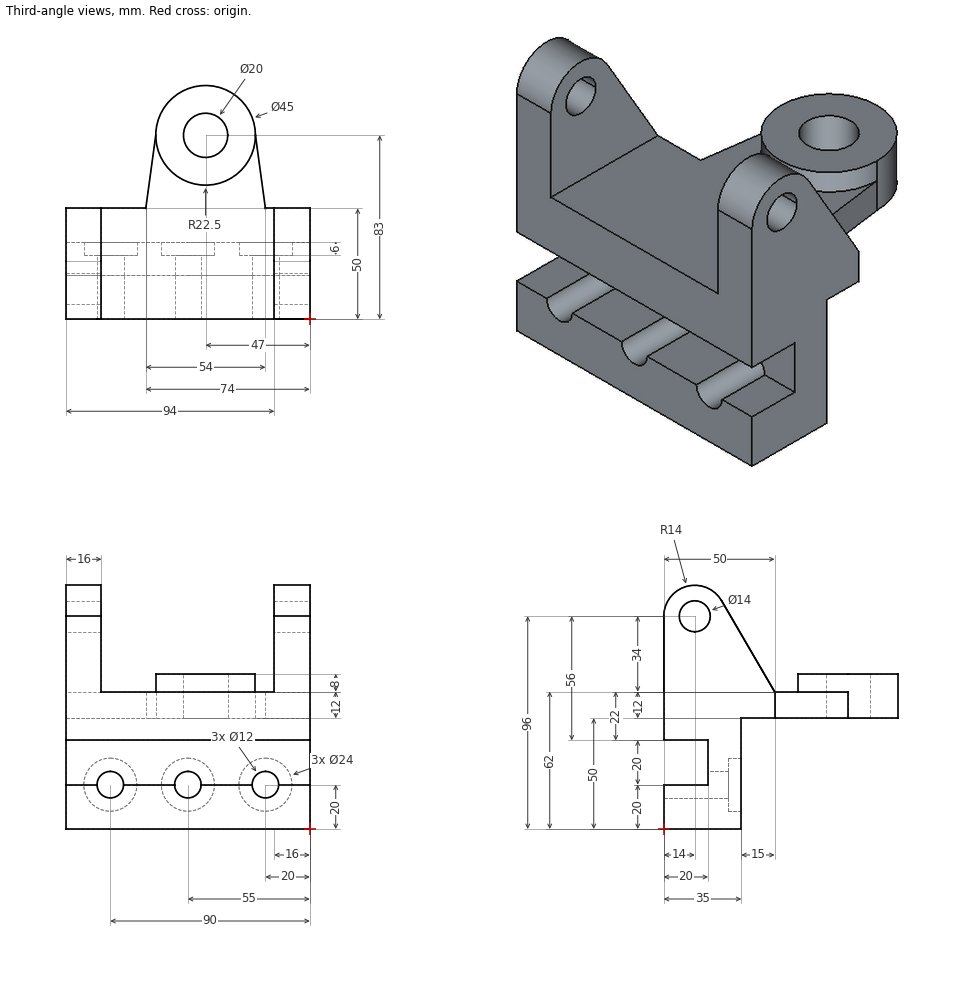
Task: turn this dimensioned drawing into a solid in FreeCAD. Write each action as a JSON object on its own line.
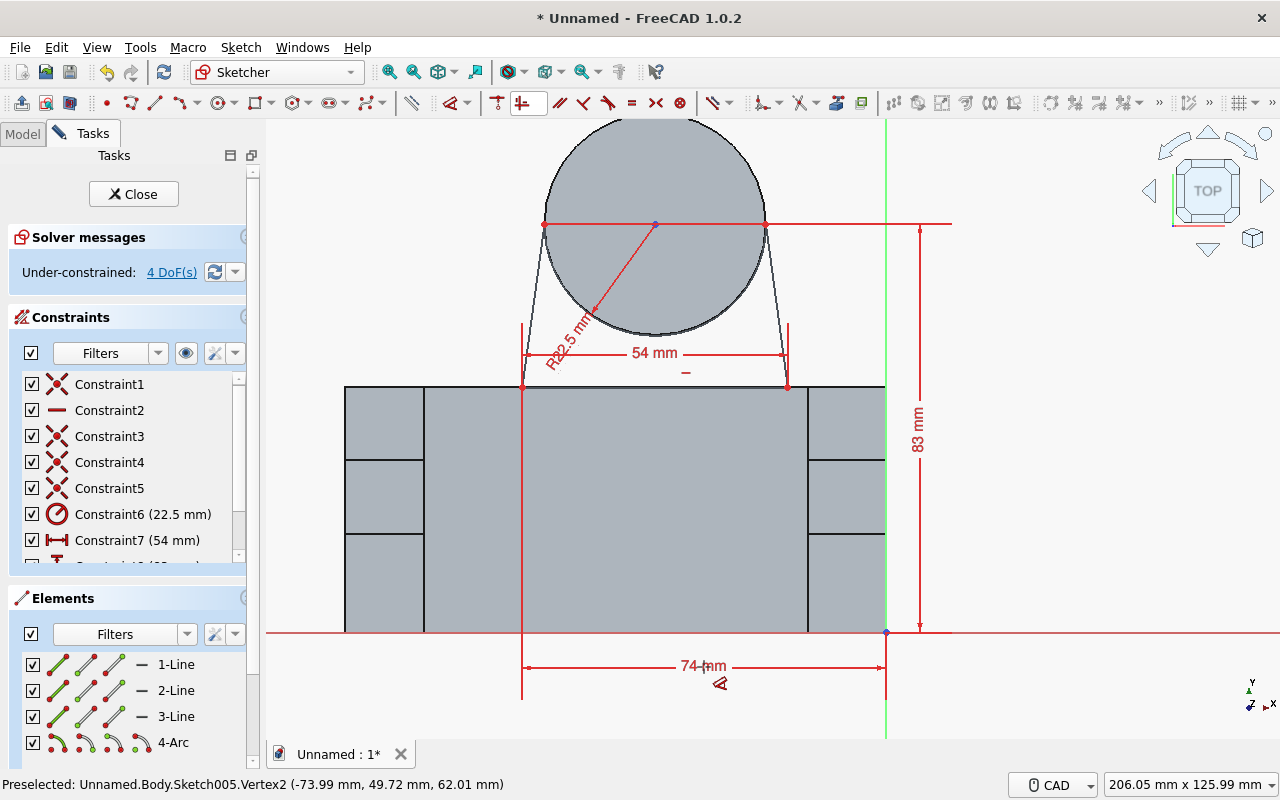
{"action": "left_click", "coordinate": [522, 388]}
{"action": "left_click", "coordinate": [920, 510]}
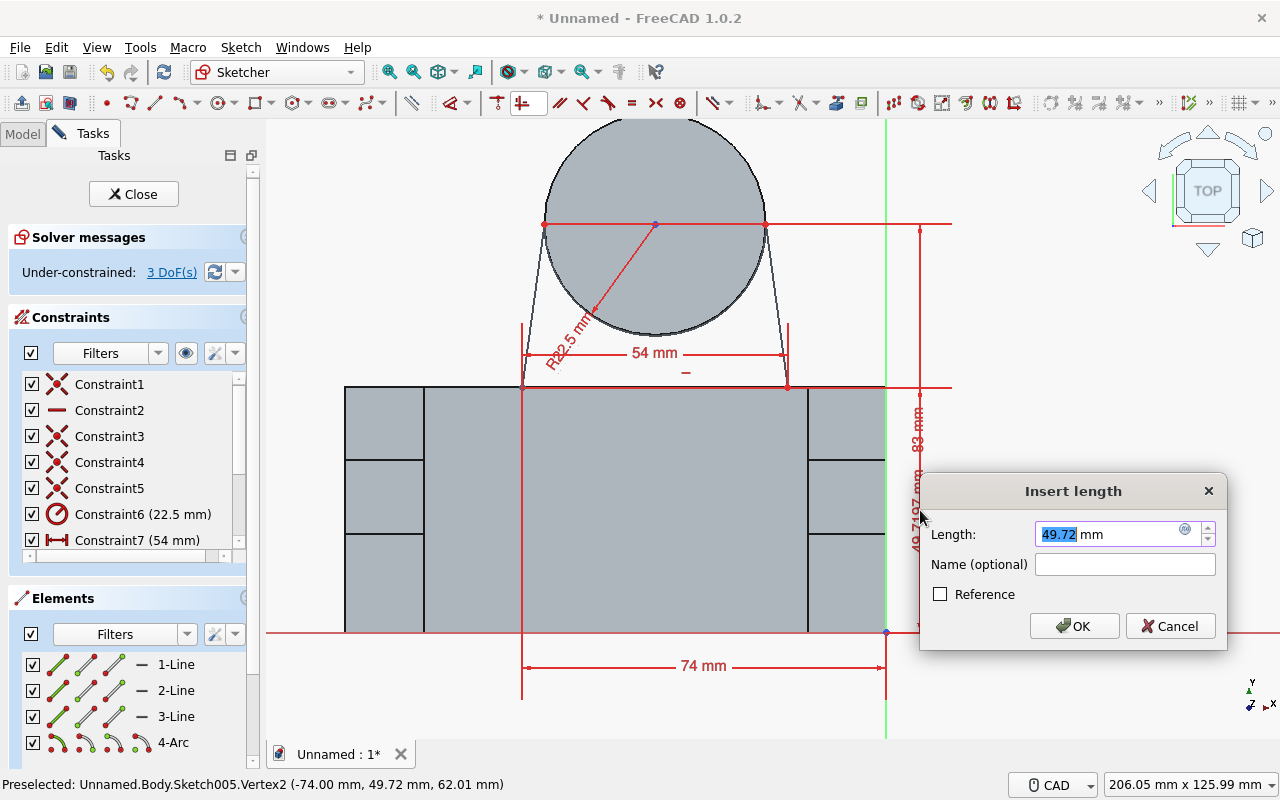
{"action": "type", "text": "50"}
{"action": "key", "text": "Return"}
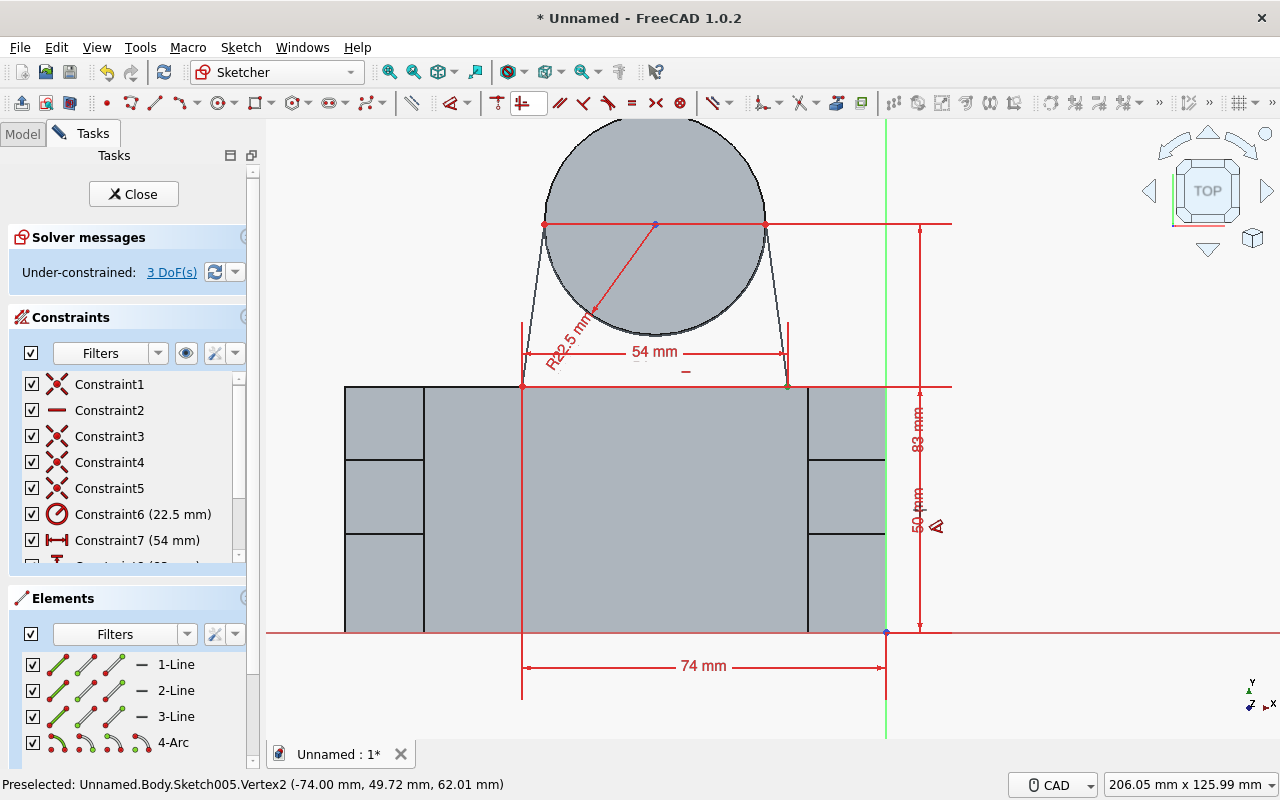
{"action": "left_click", "coordinate": [766, 225]}
{"action": "left_click", "coordinate": [920, 335]}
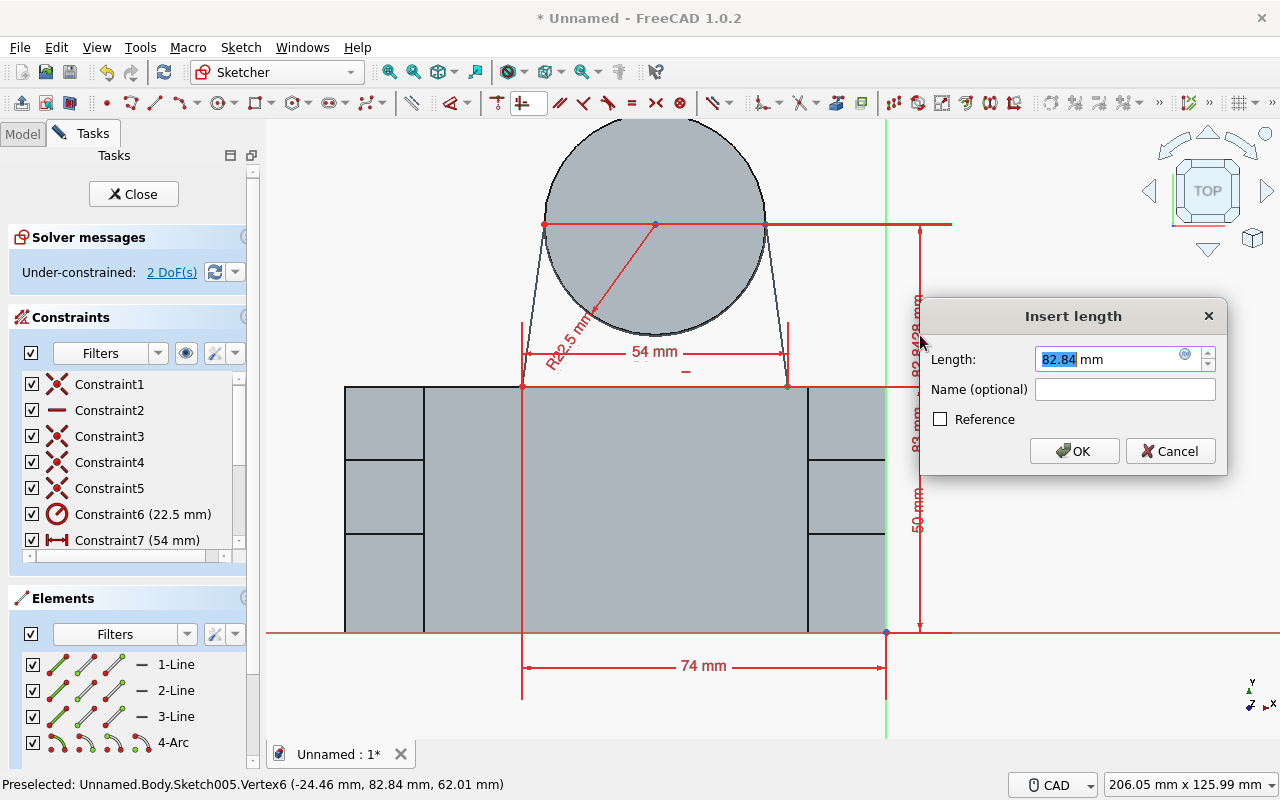
{"action": "type", "text": "83"}
{"action": "key", "text": "Return"}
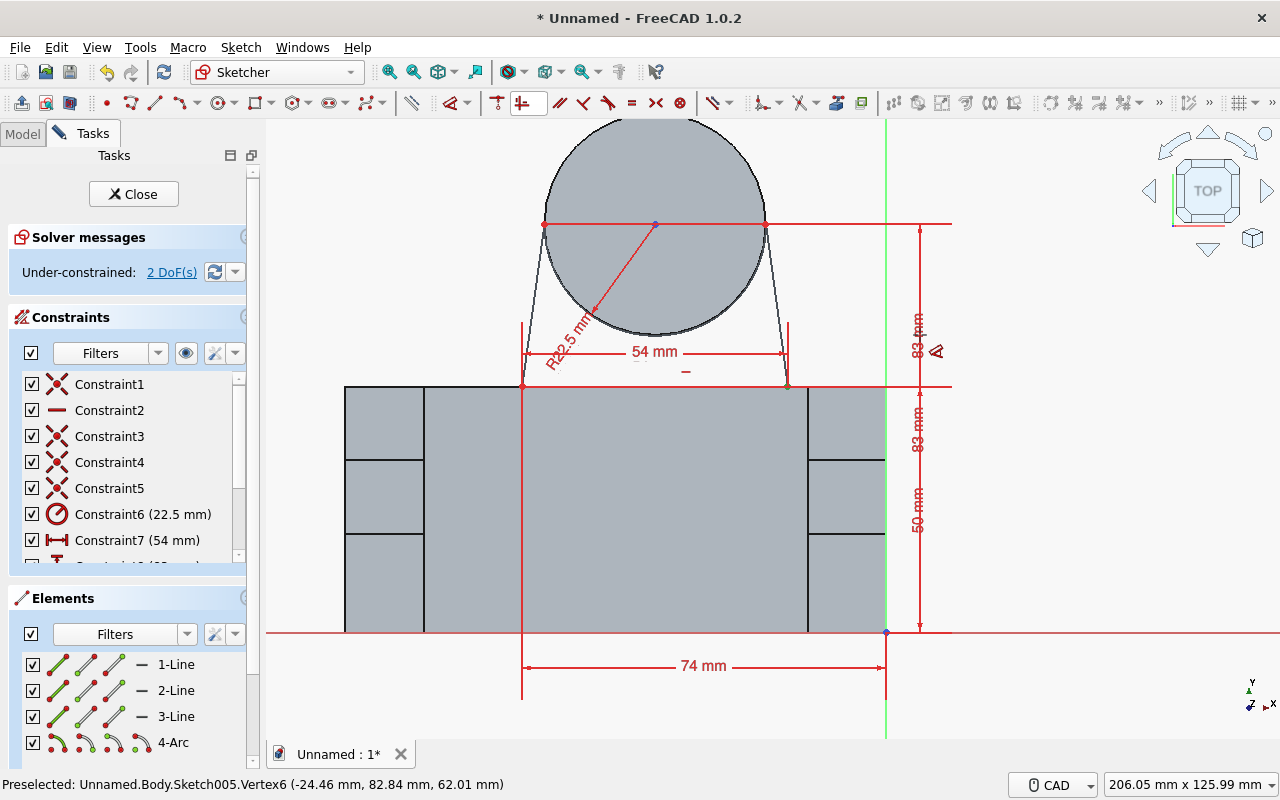
{"action": "left_click", "coordinate": [655, 225]}
{"action": "left_click", "coordinate": [824, 667]}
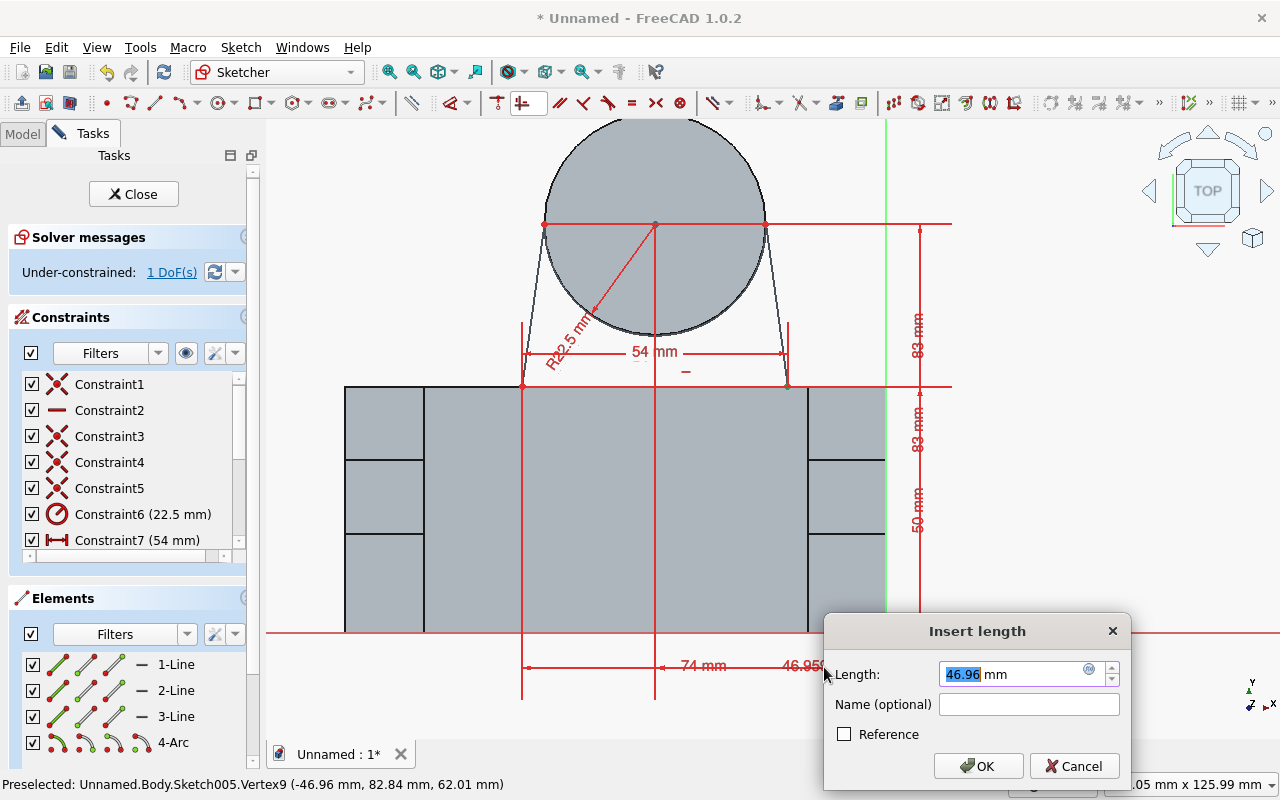
{"action": "type", "text": "47"}
{"action": "key", "text": "Return"}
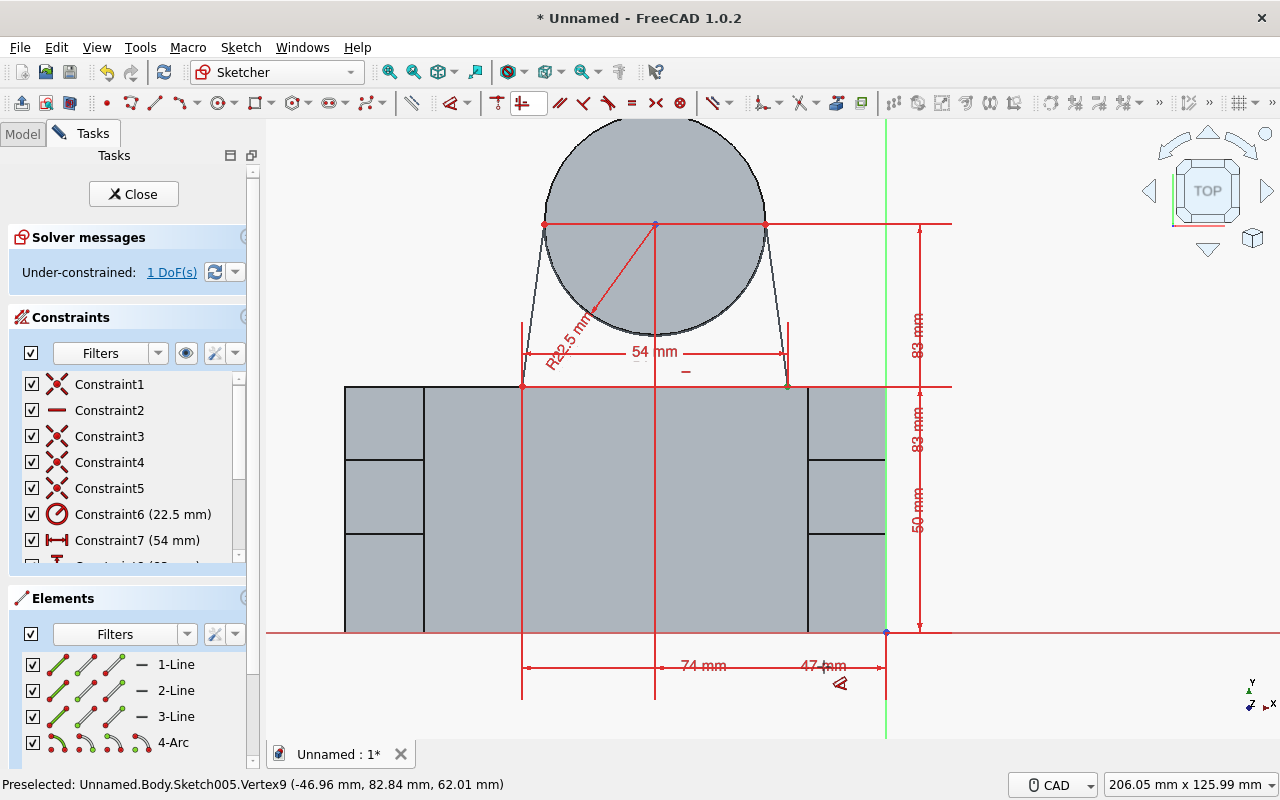
{"action": "left_click", "coordinate": [655, 225]}
{"action": "left_click", "coordinate": [920, 286]}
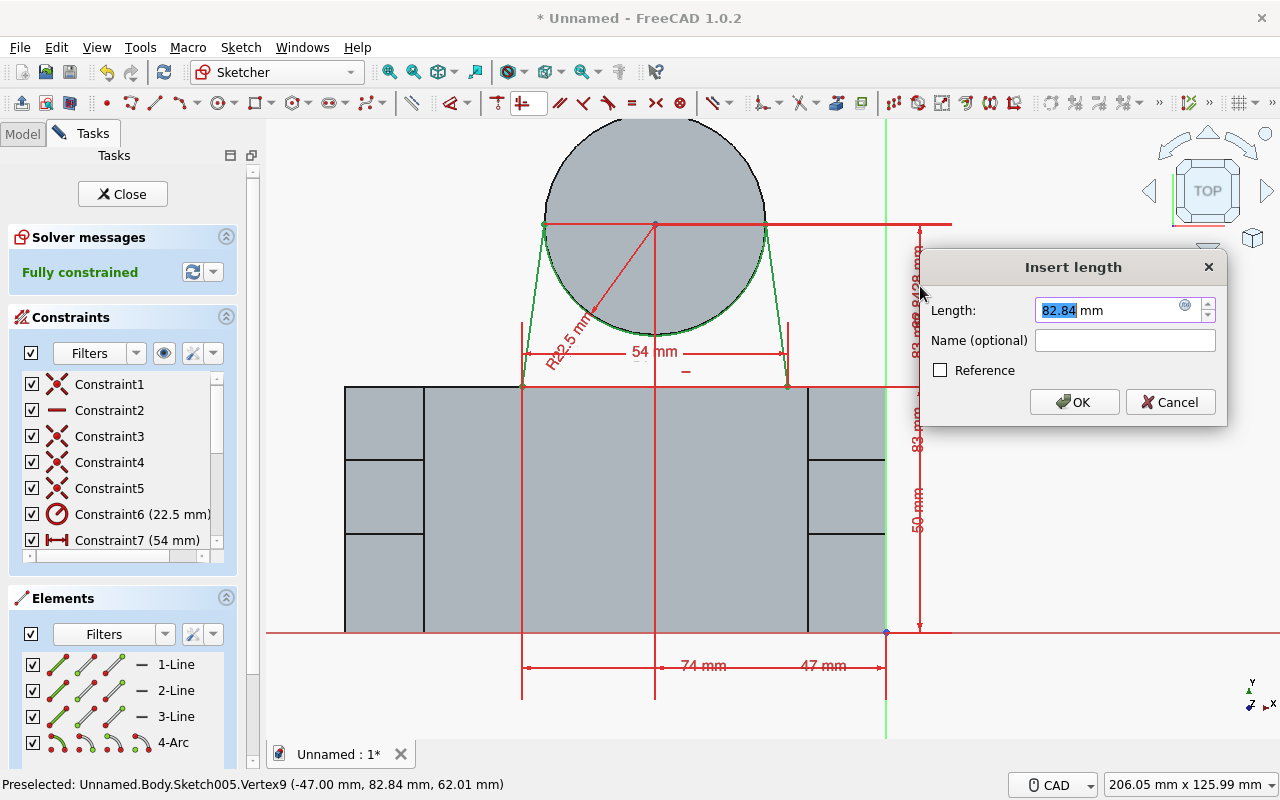
{"action": "type", "text": "83"}
{"action": "key", "text": "Return"}
{"action": "key", "text": "Escape"}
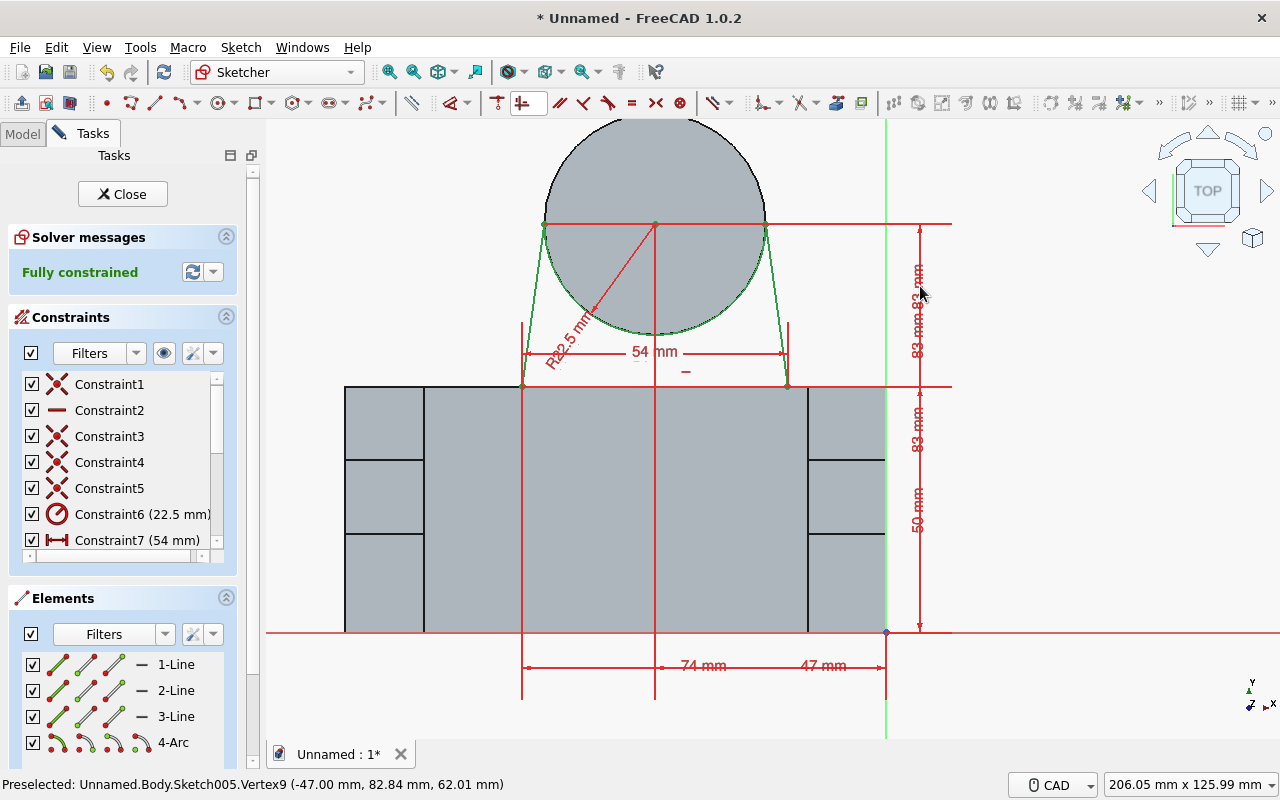
{"action": "left_click", "coordinate": [123, 194]}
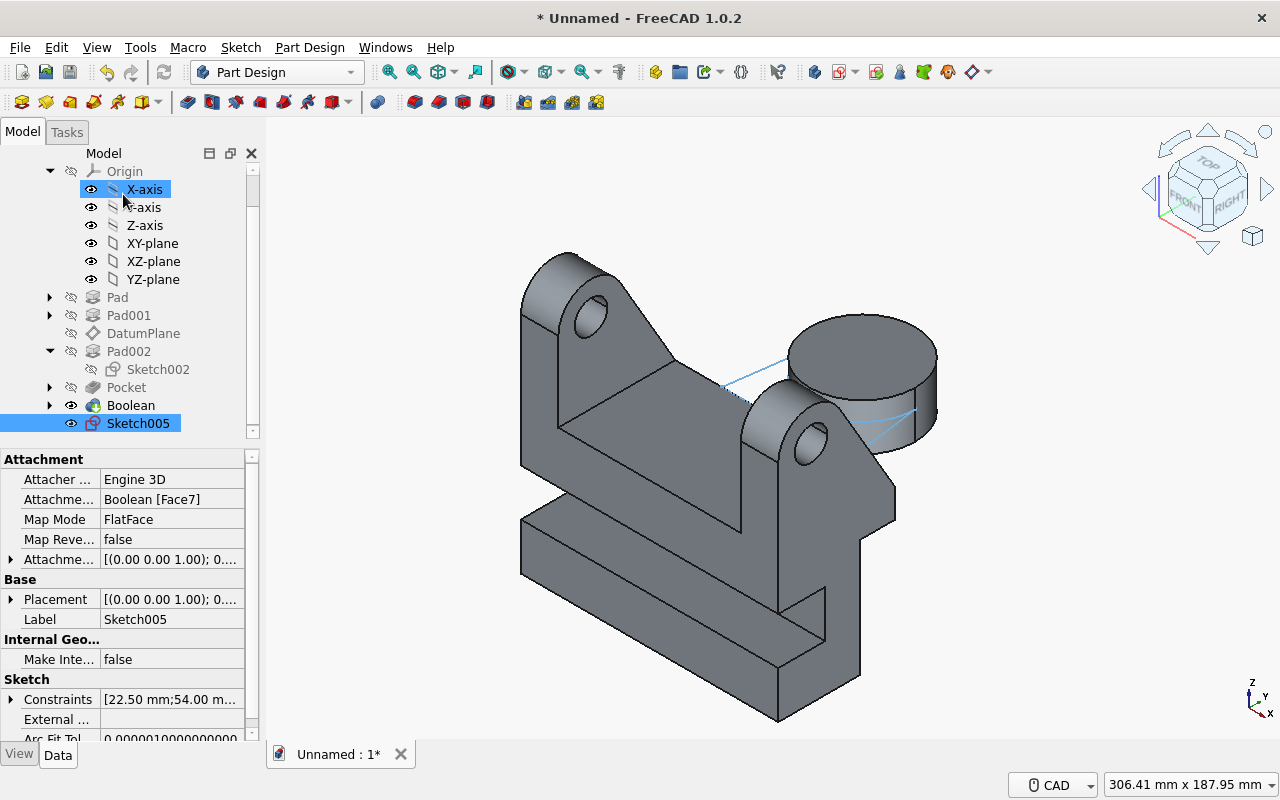
{"action": "left_click", "coordinate": [22, 102]}